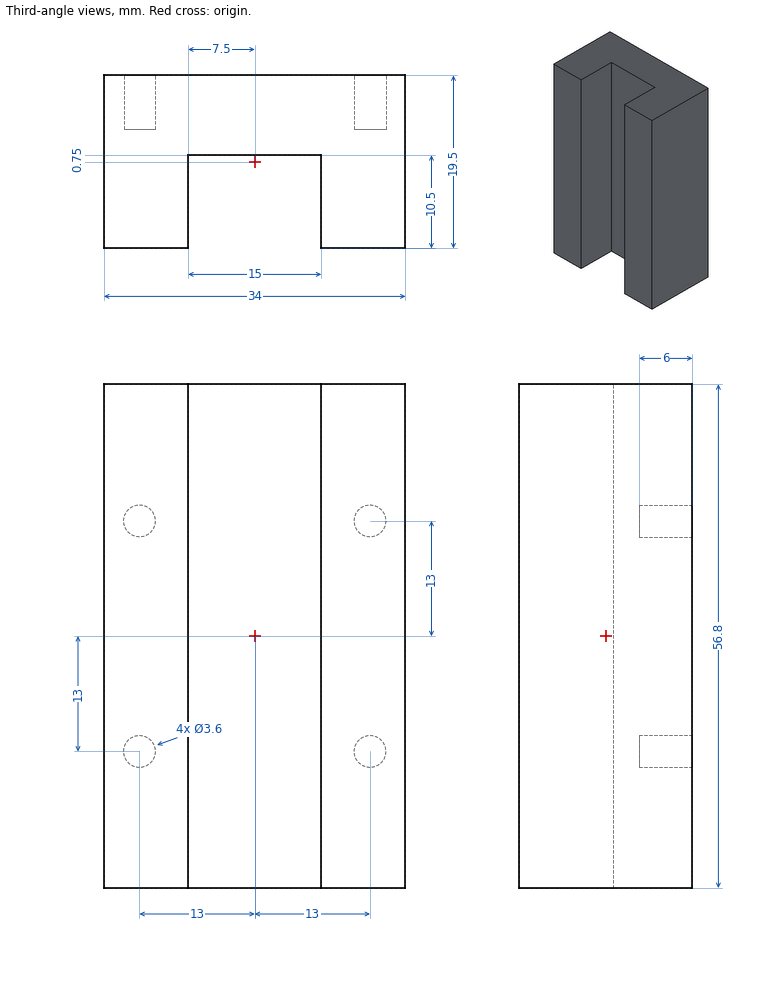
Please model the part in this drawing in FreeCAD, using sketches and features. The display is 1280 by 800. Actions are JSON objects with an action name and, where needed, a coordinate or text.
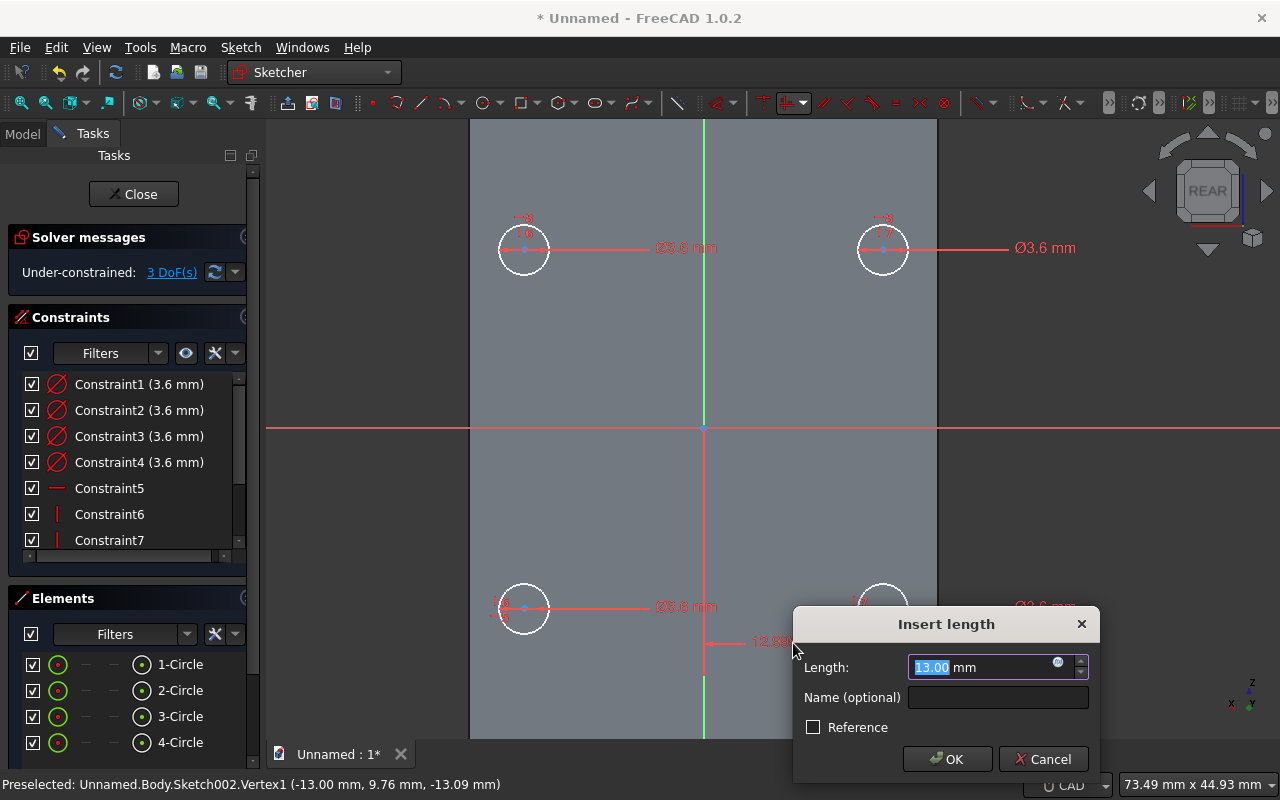
{"action": "type", "text": "13"}
{"action": "key", "text": "Return"}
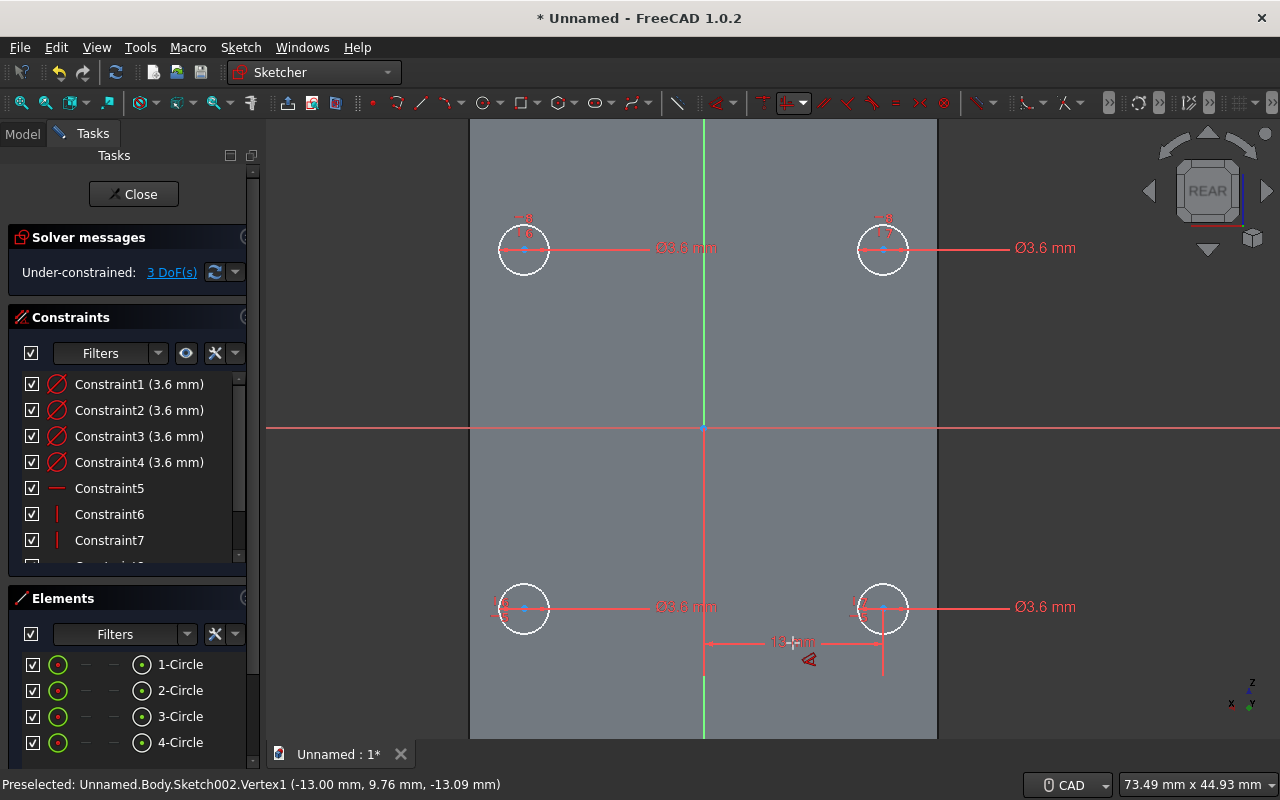
{"action": "left_click", "coordinate": [883, 609]}
{"action": "left_click", "coordinate": [917, 519]}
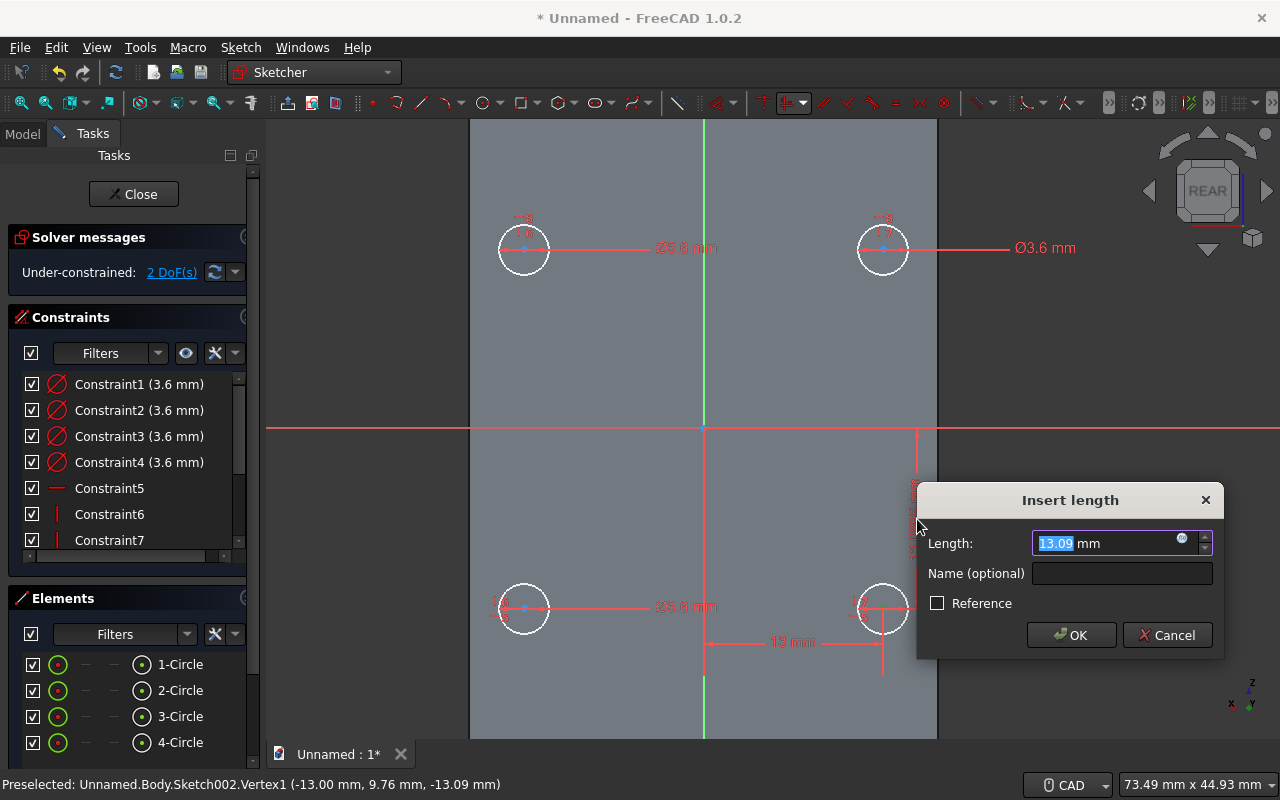
{"action": "type", "text": "13"}
{"action": "key", "text": "Return"}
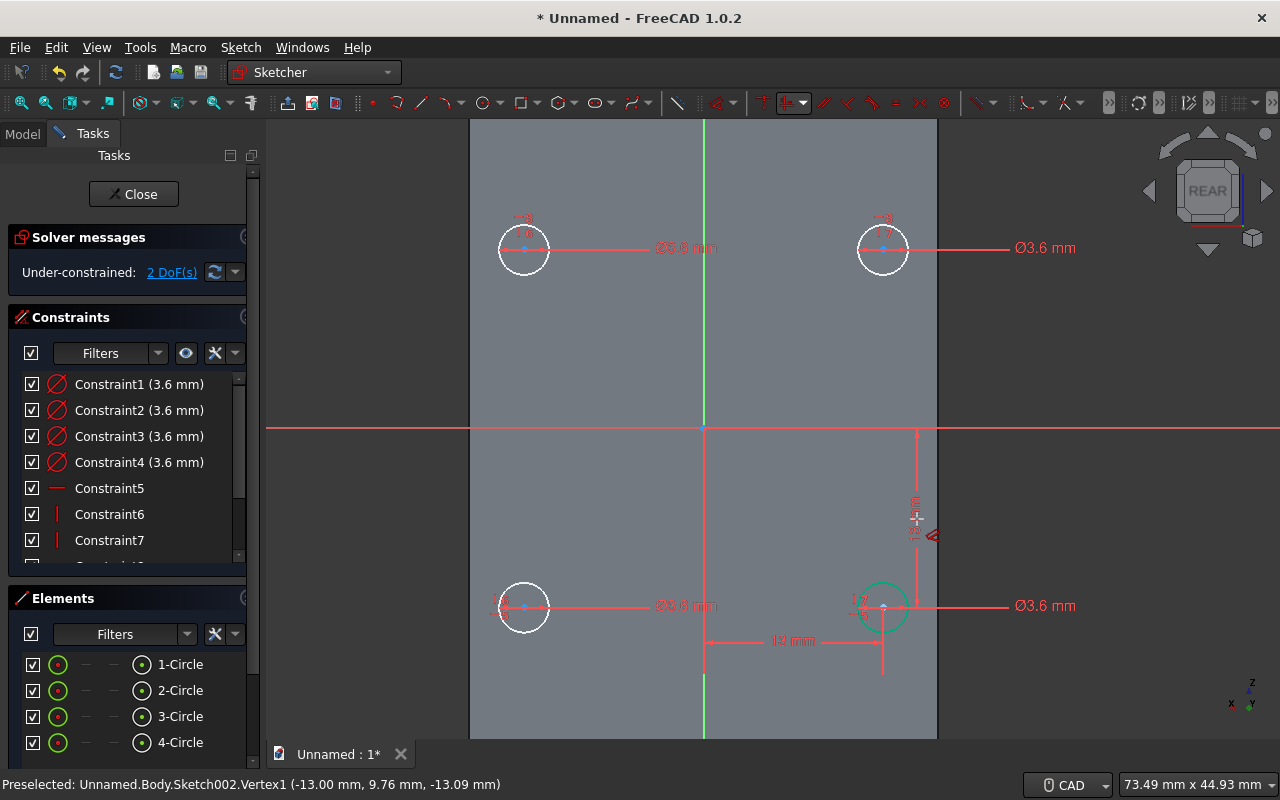
{"action": "left_click", "coordinate": [524, 608]}
{"action": "left_click", "coordinate": [614, 642]}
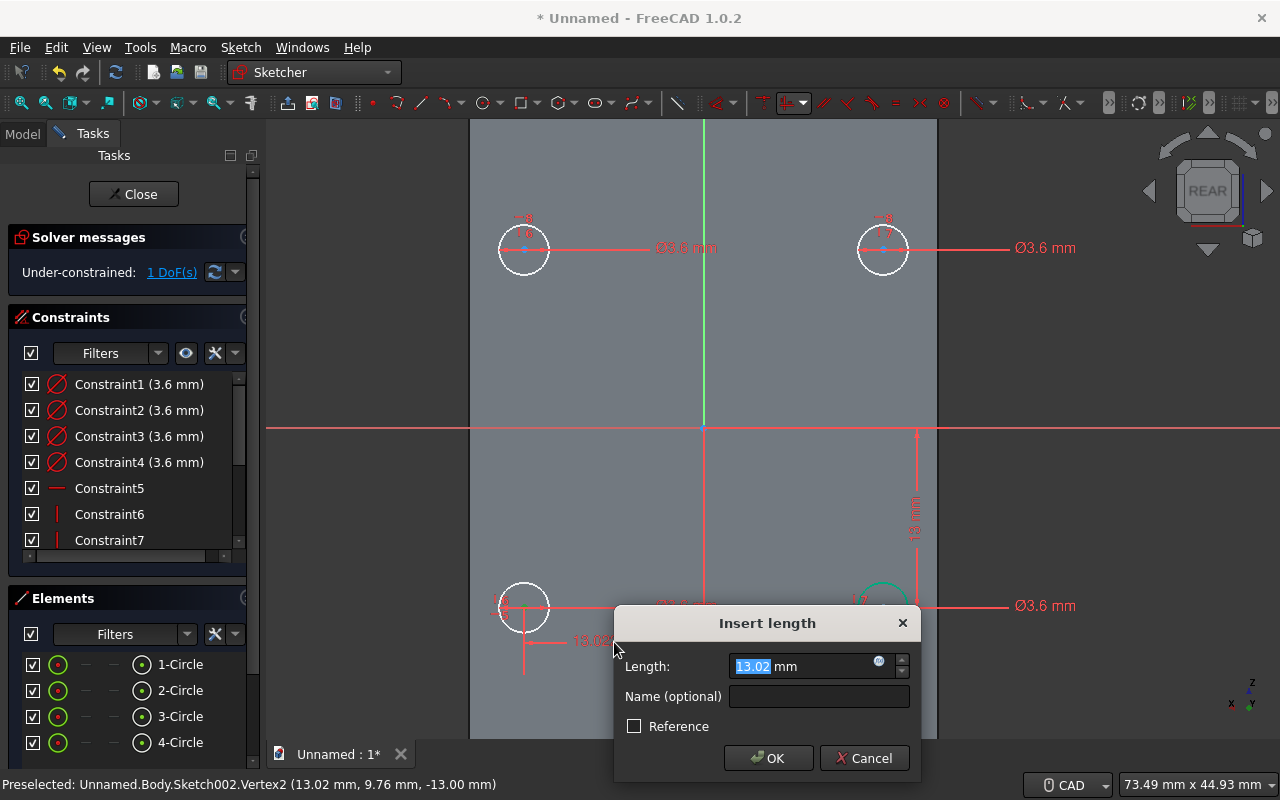
{"action": "type", "text": "13"}
{"action": "key", "text": "Return"}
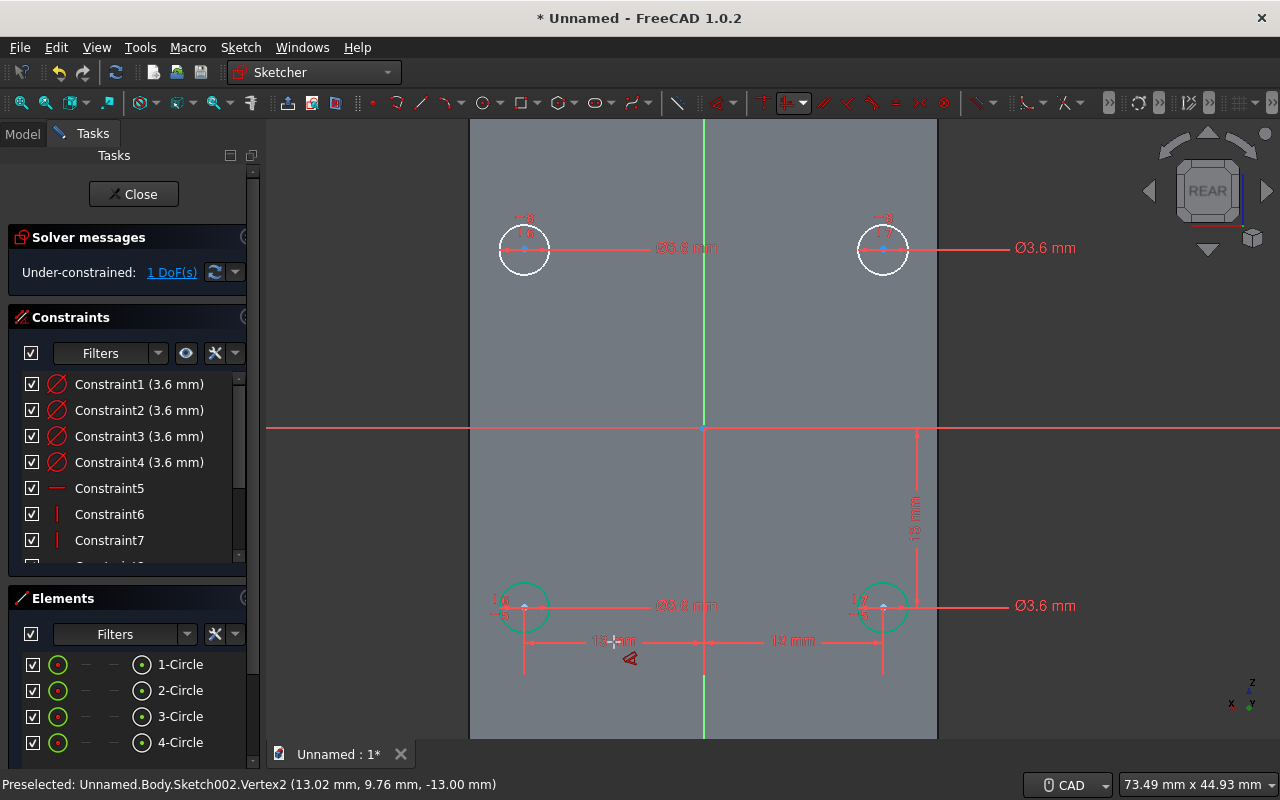
{"action": "left_click", "coordinate": [524, 250]}
{"action": "left_click", "coordinate": [490, 339]}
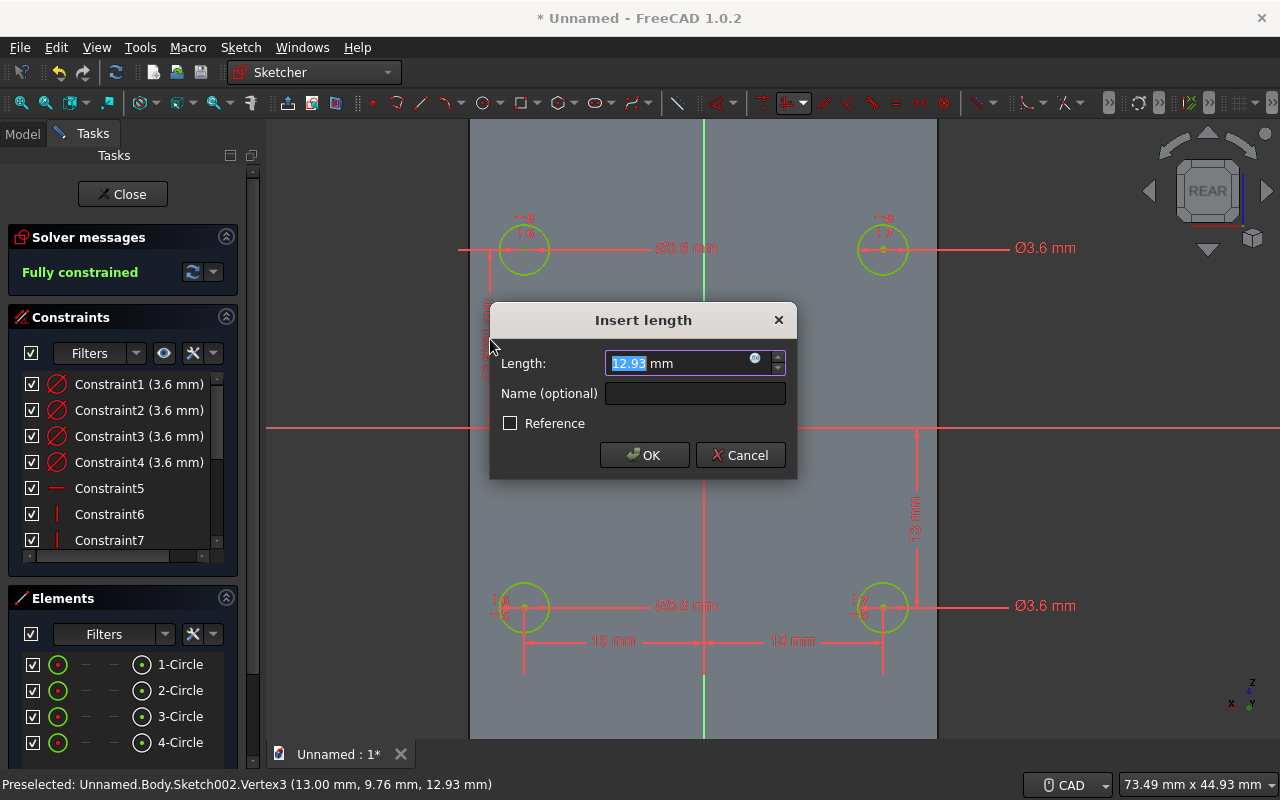
{"action": "type", "text": "13"}
{"action": "key", "text": "Return"}
{"action": "key", "text": "Escape"}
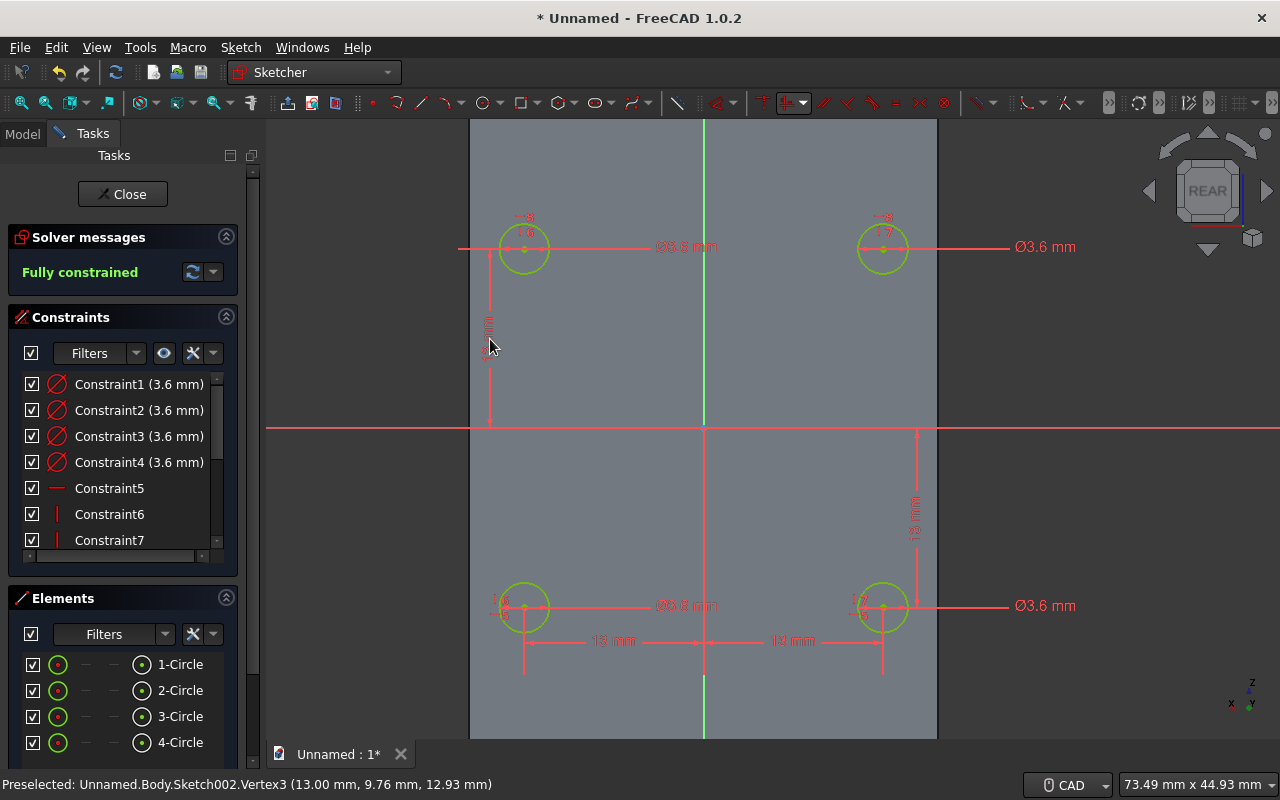
{"action": "left_click", "coordinate": [123, 194]}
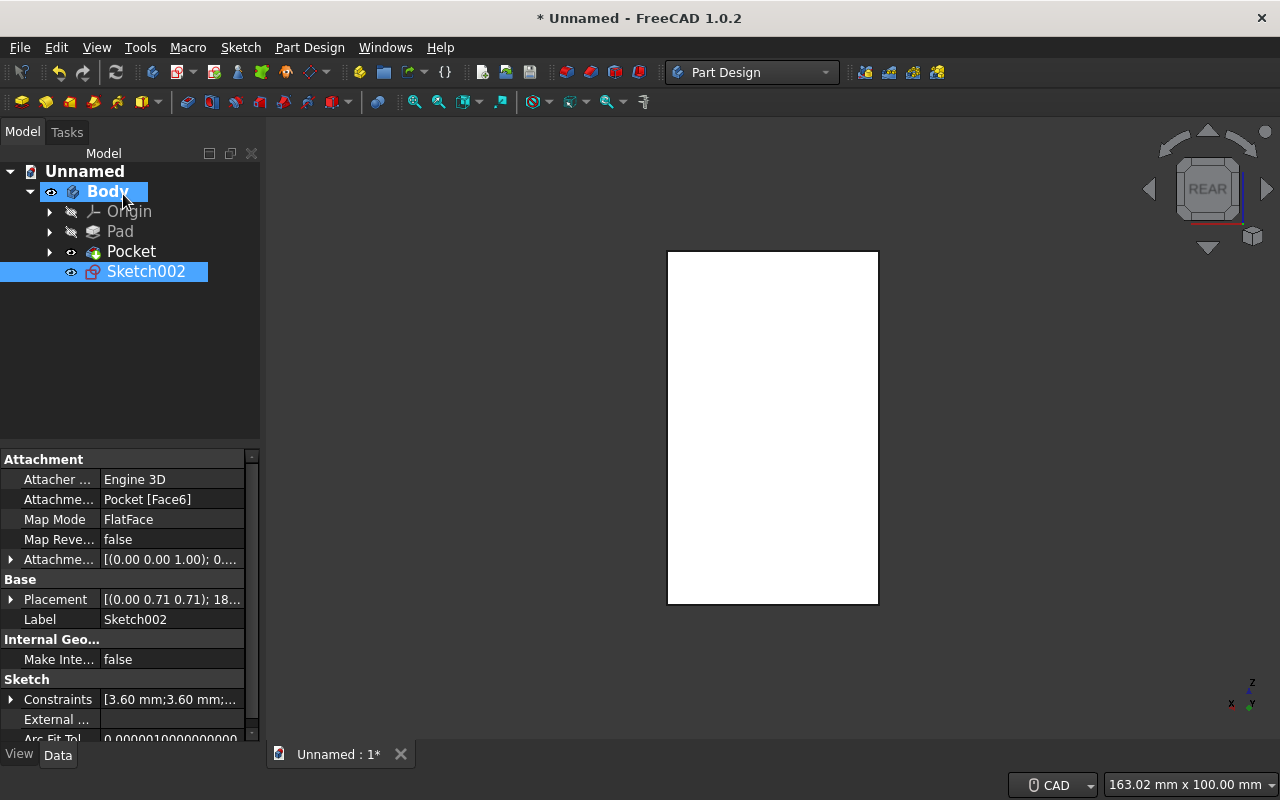
{"action": "left_click", "coordinate": [188, 102]}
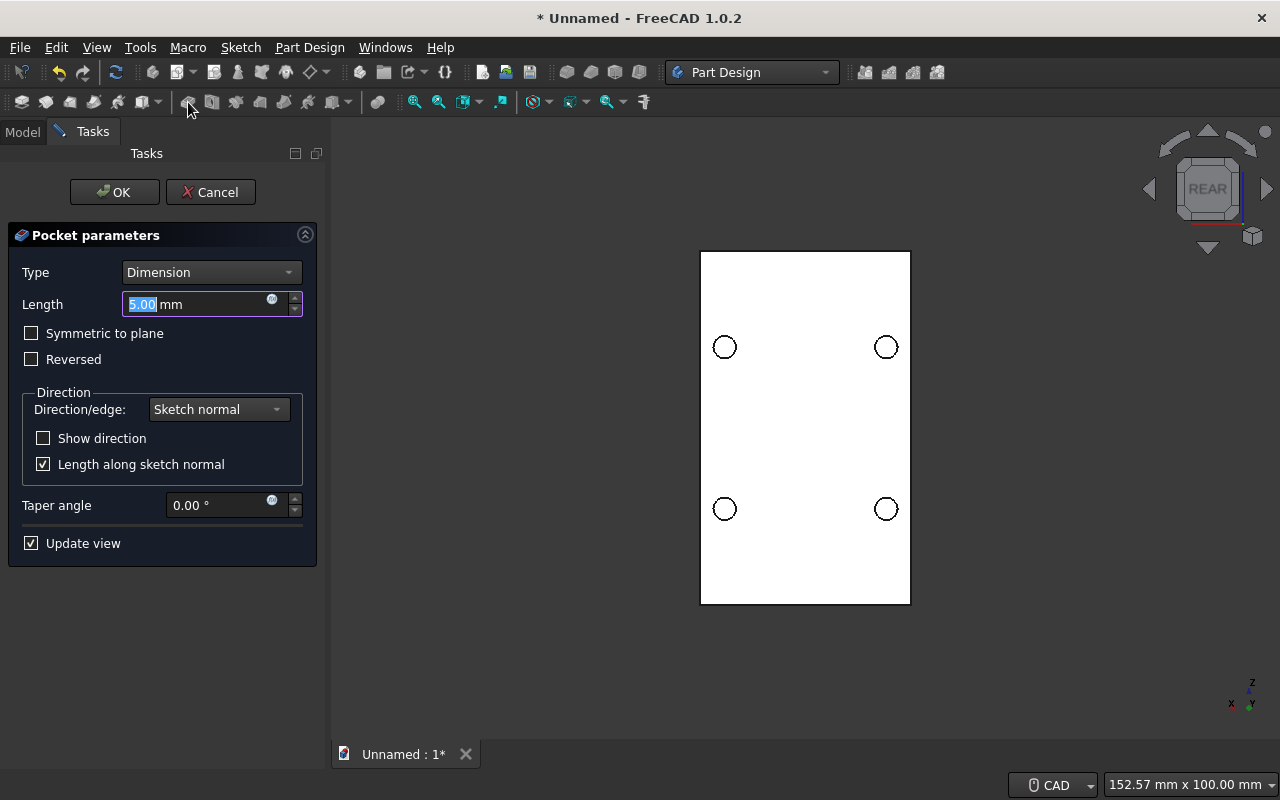
{"action": "type", "text": "6"}
{"action": "key", "text": "Tab"}